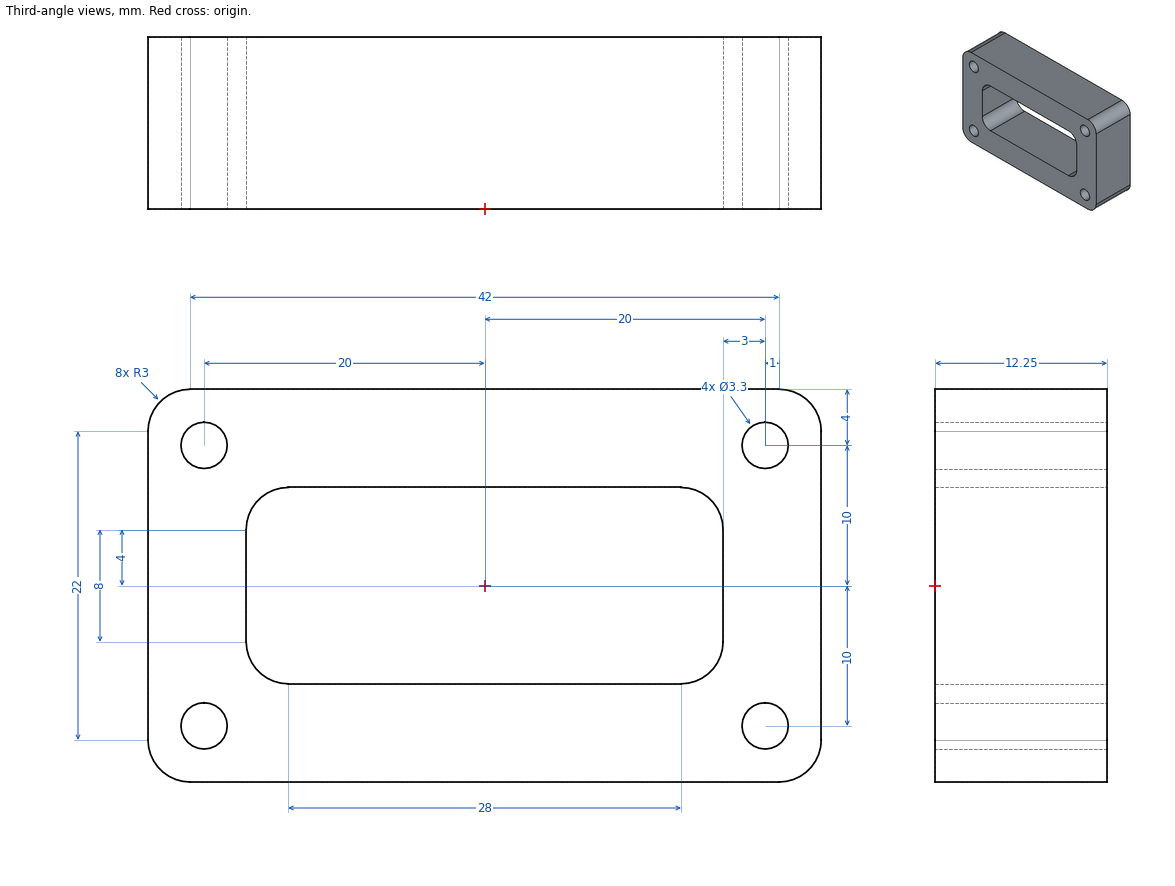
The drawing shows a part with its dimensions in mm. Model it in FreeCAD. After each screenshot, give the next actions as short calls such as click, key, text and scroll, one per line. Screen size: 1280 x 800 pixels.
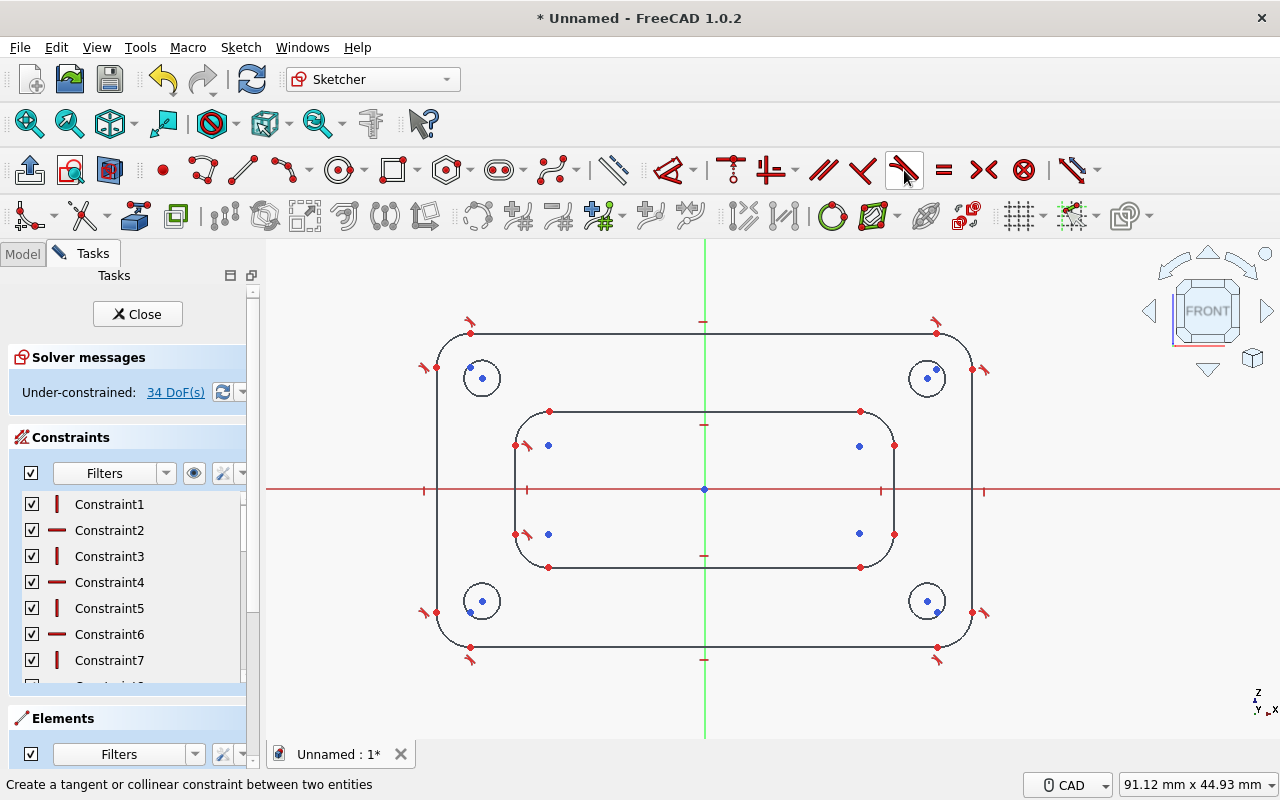
click(642, 568)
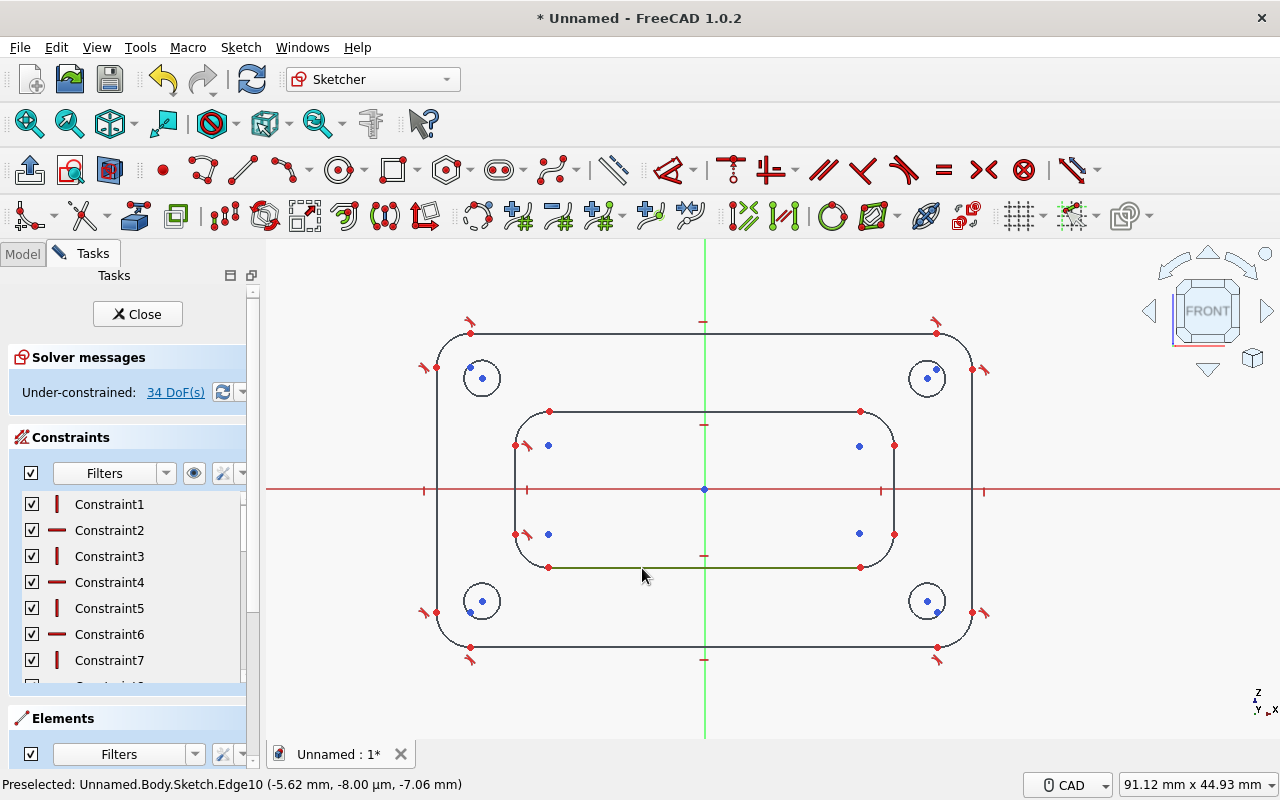
click(519, 550)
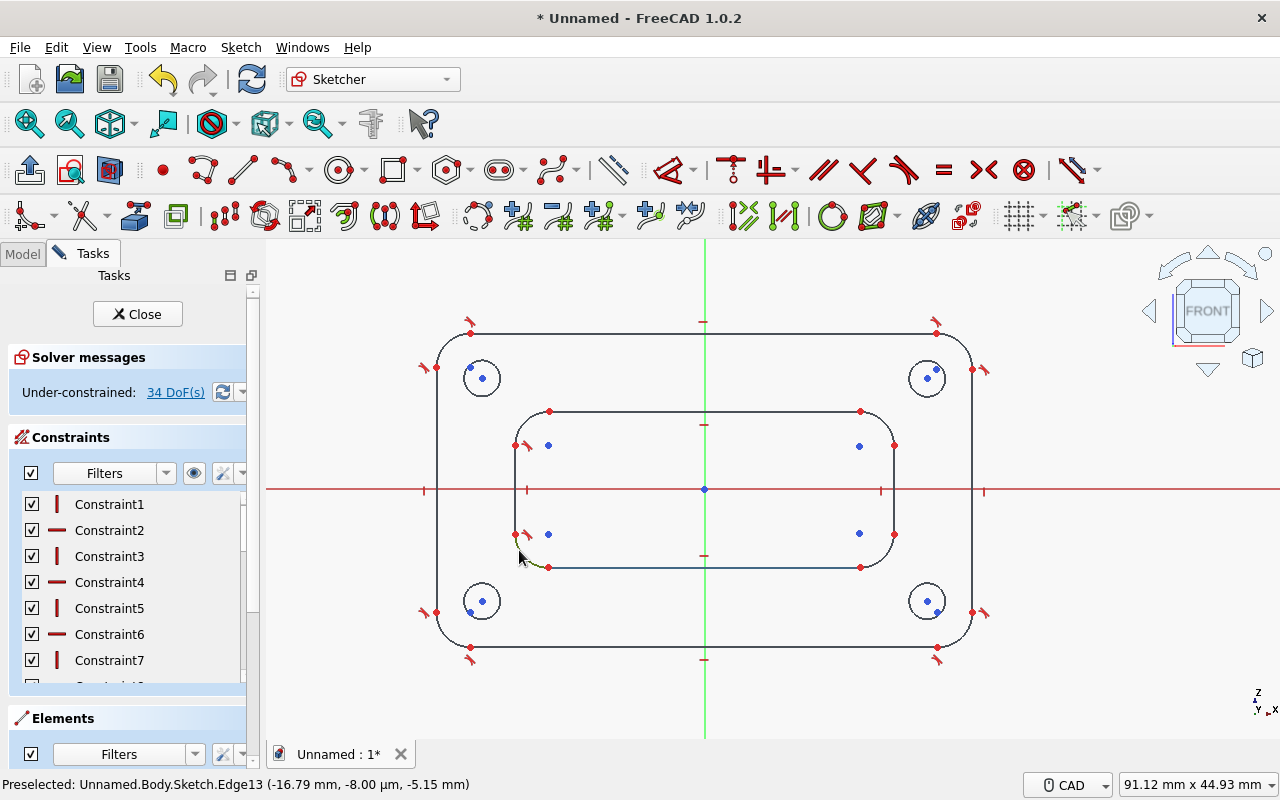
click(904, 170)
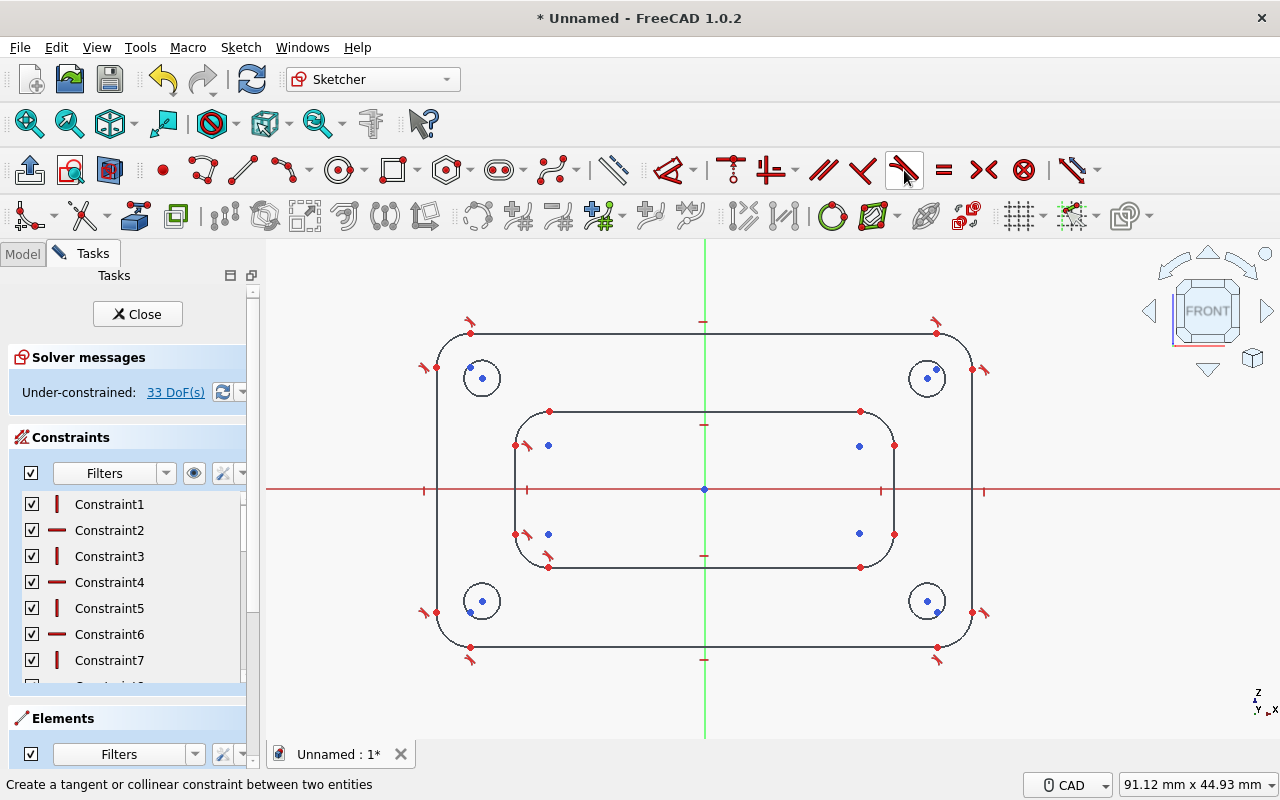
click(642, 568)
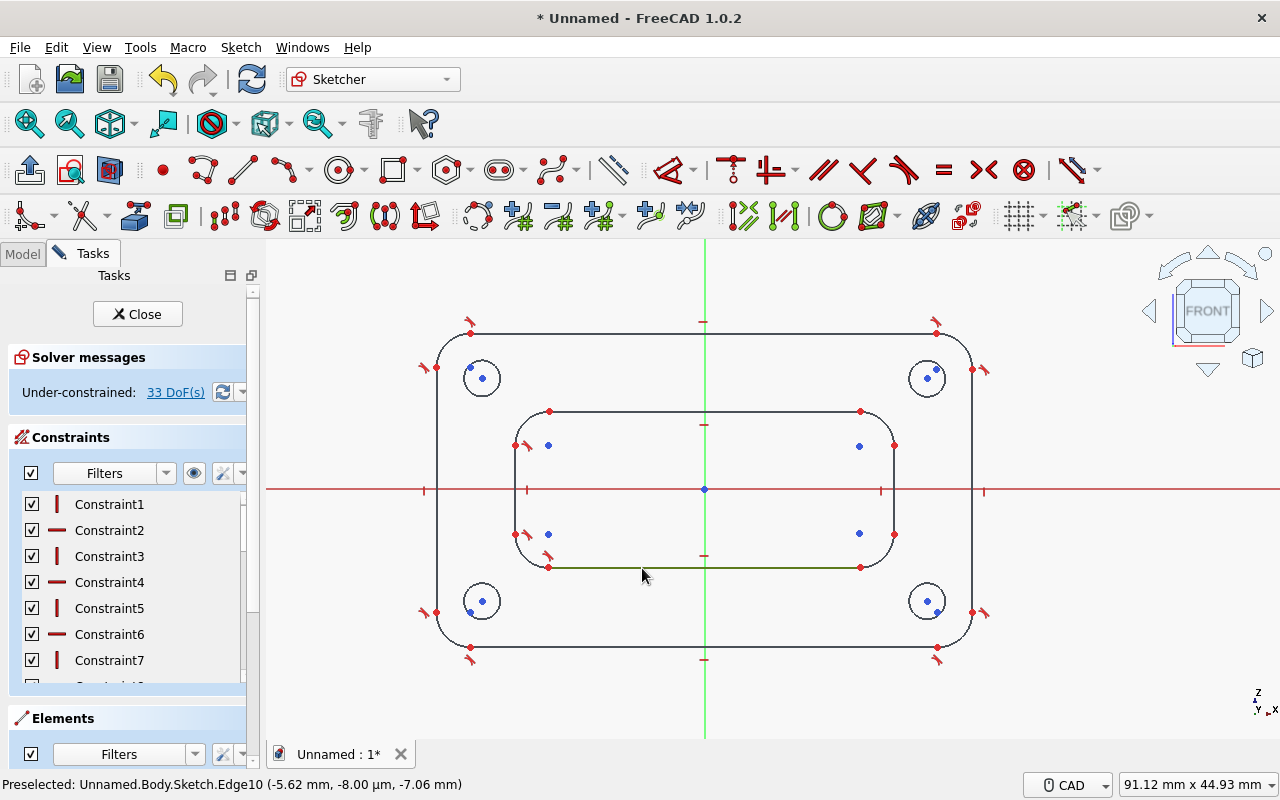
click(875, 564)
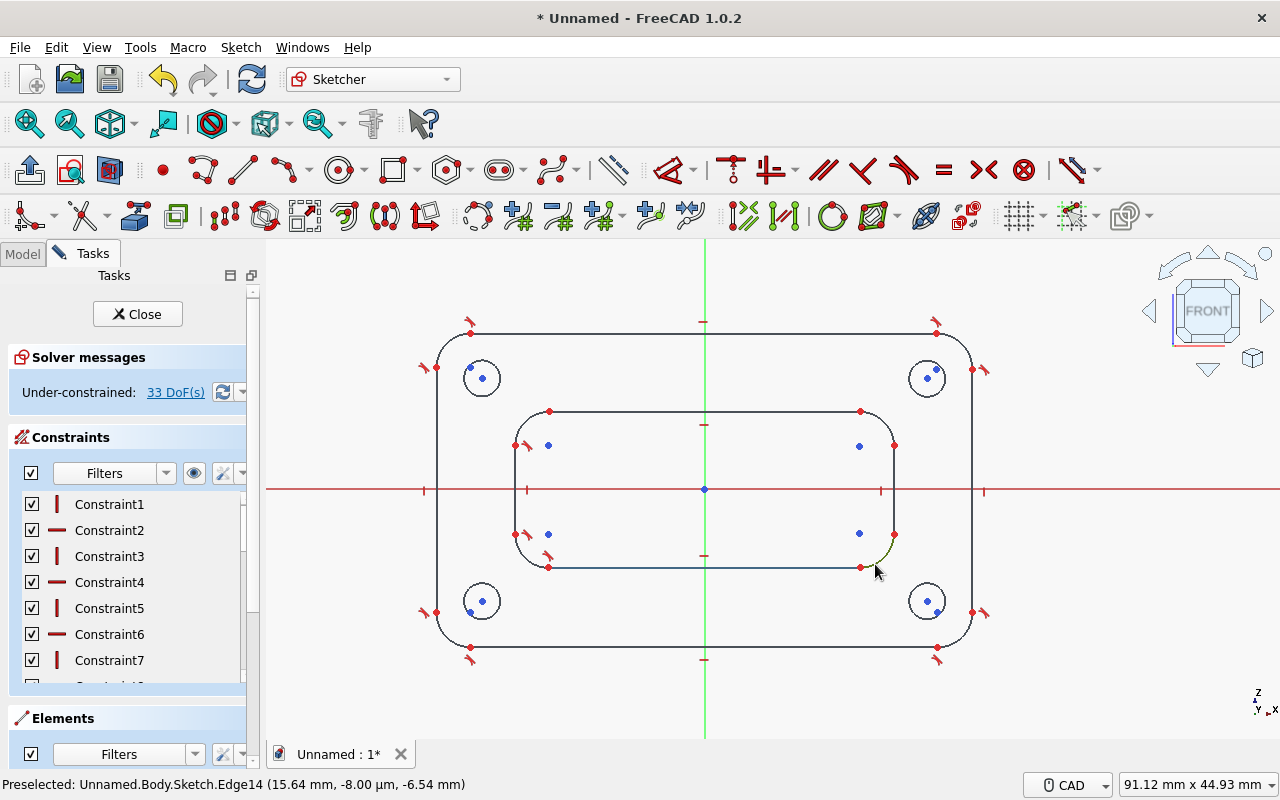
click(904, 170)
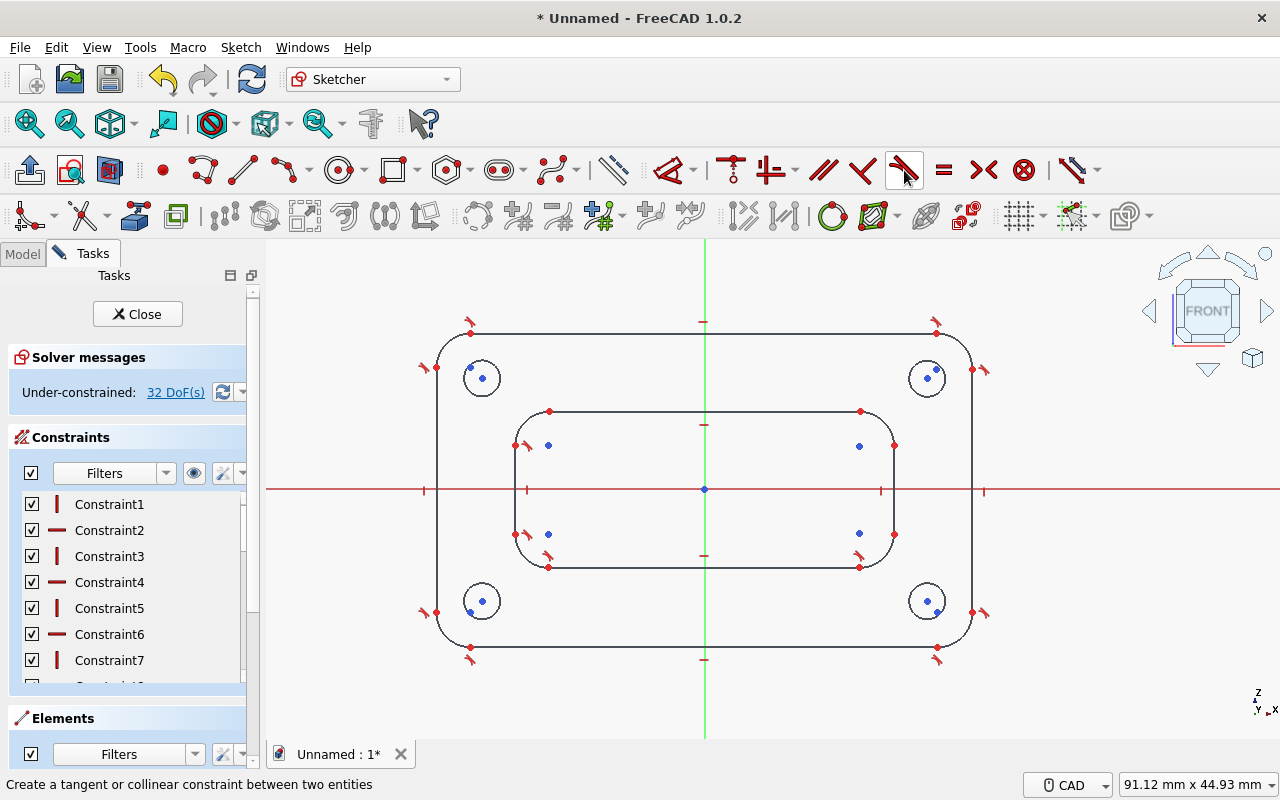
click(894, 508)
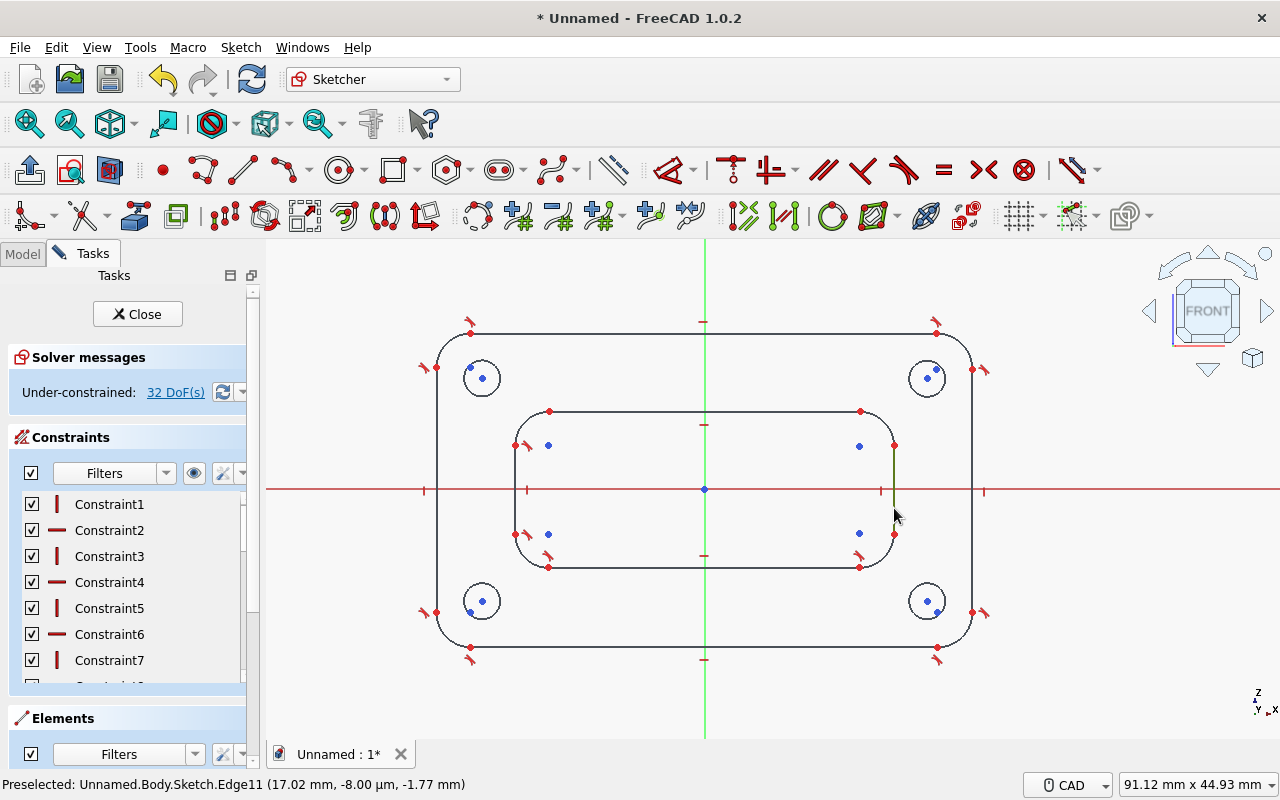
click(875, 564)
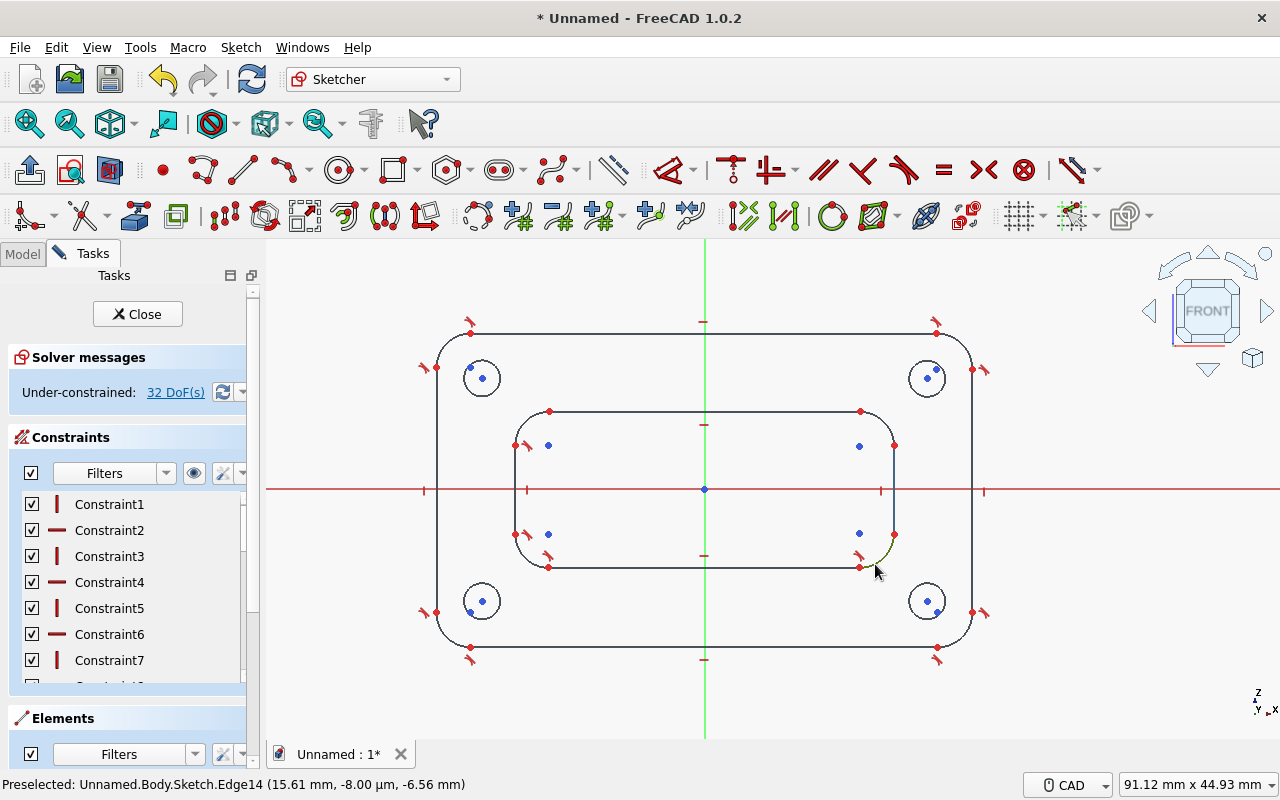
click(904, 170)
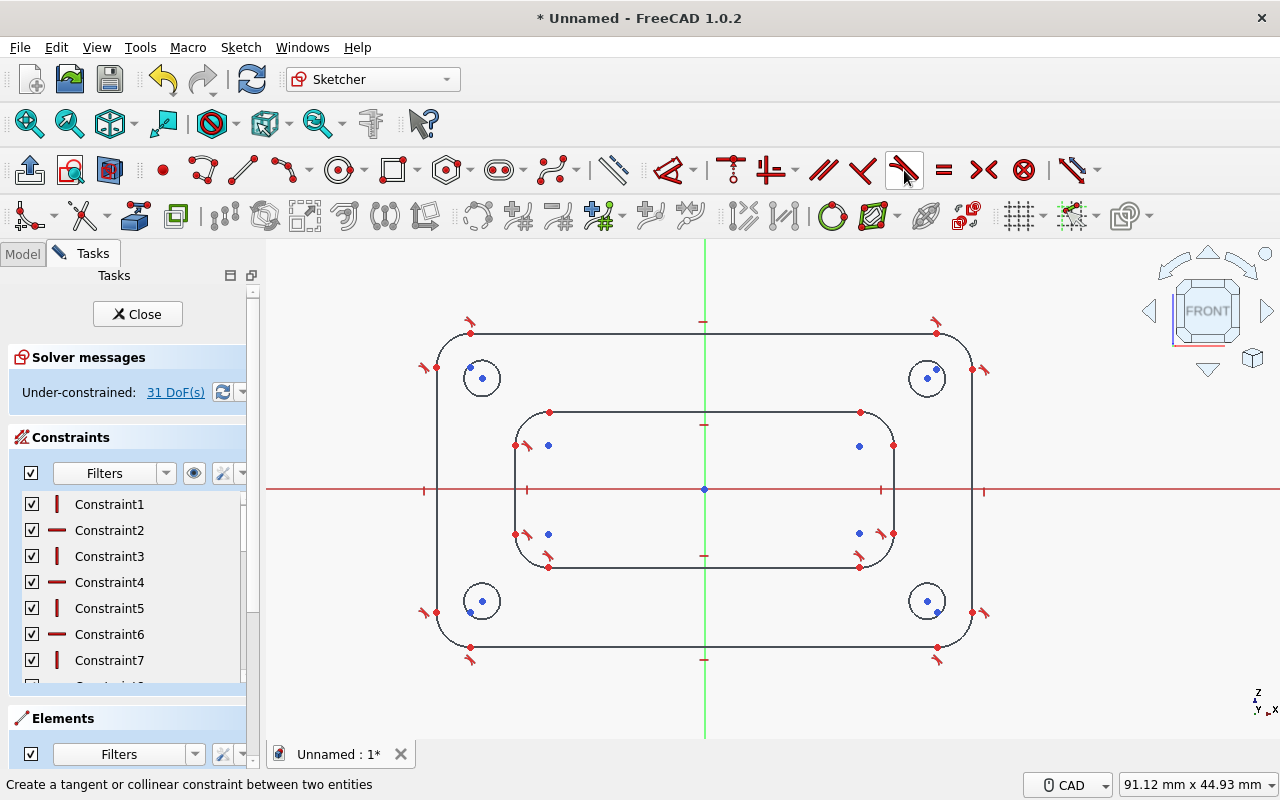
click(894, 507)